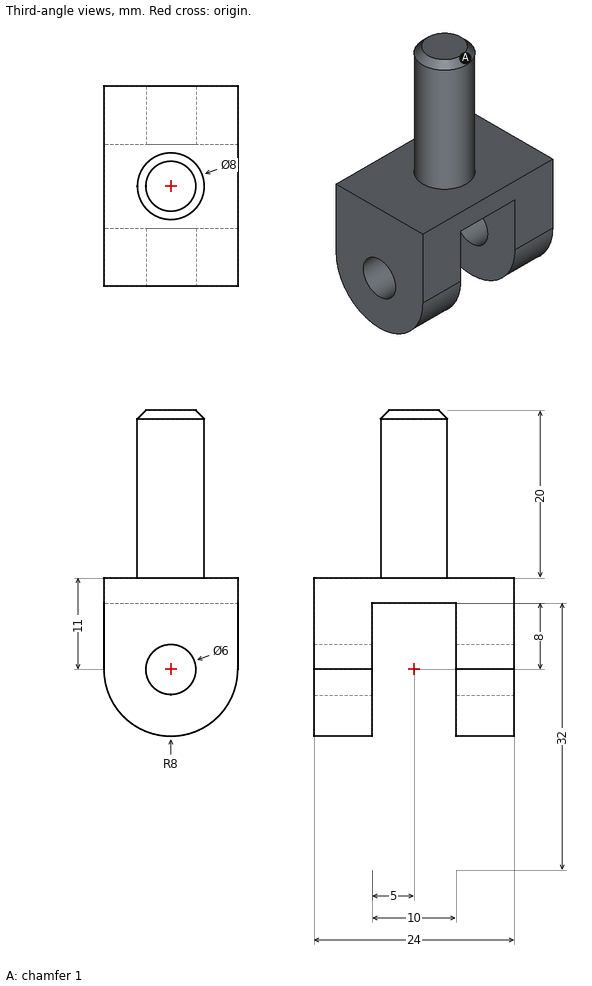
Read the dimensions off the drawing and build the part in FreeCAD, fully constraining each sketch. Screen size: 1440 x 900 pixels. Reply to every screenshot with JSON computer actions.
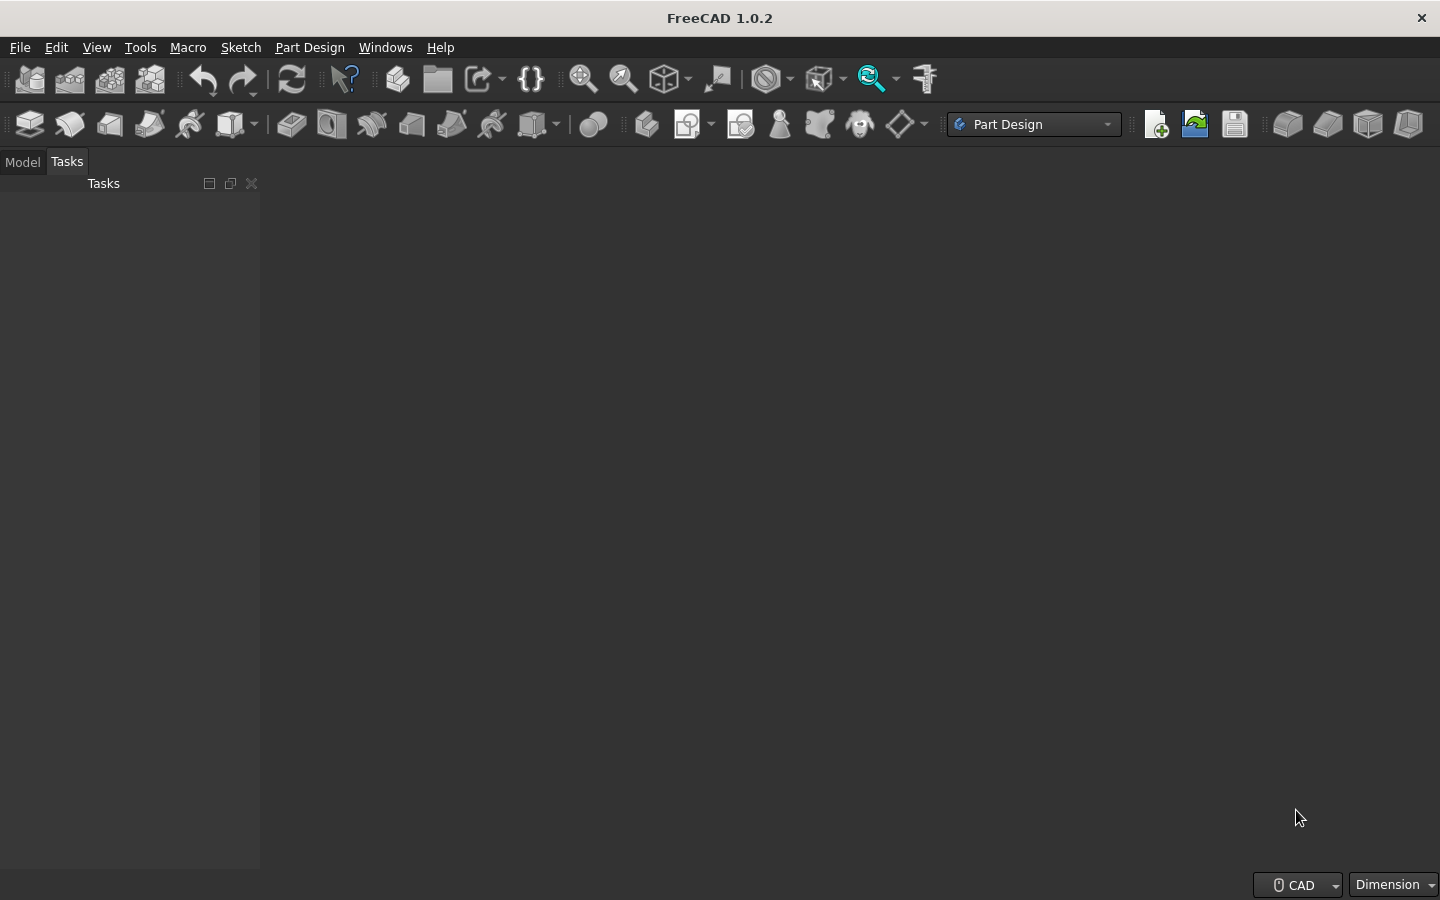
{"action": "left_click", "coordinate": [1156, 124]}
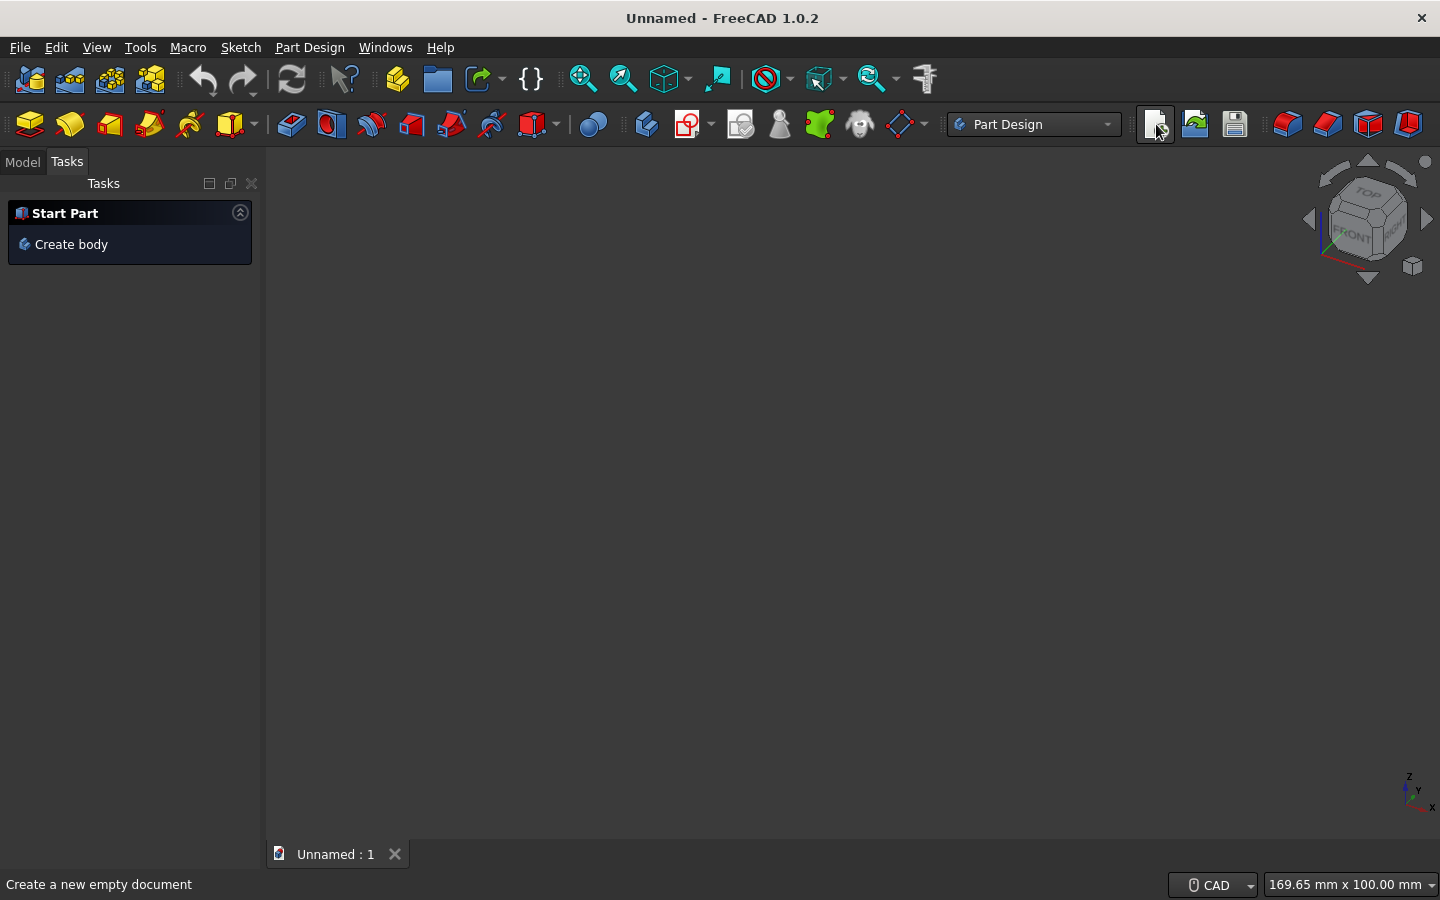
{"action": "left_click", "coordinate": [688, 124]}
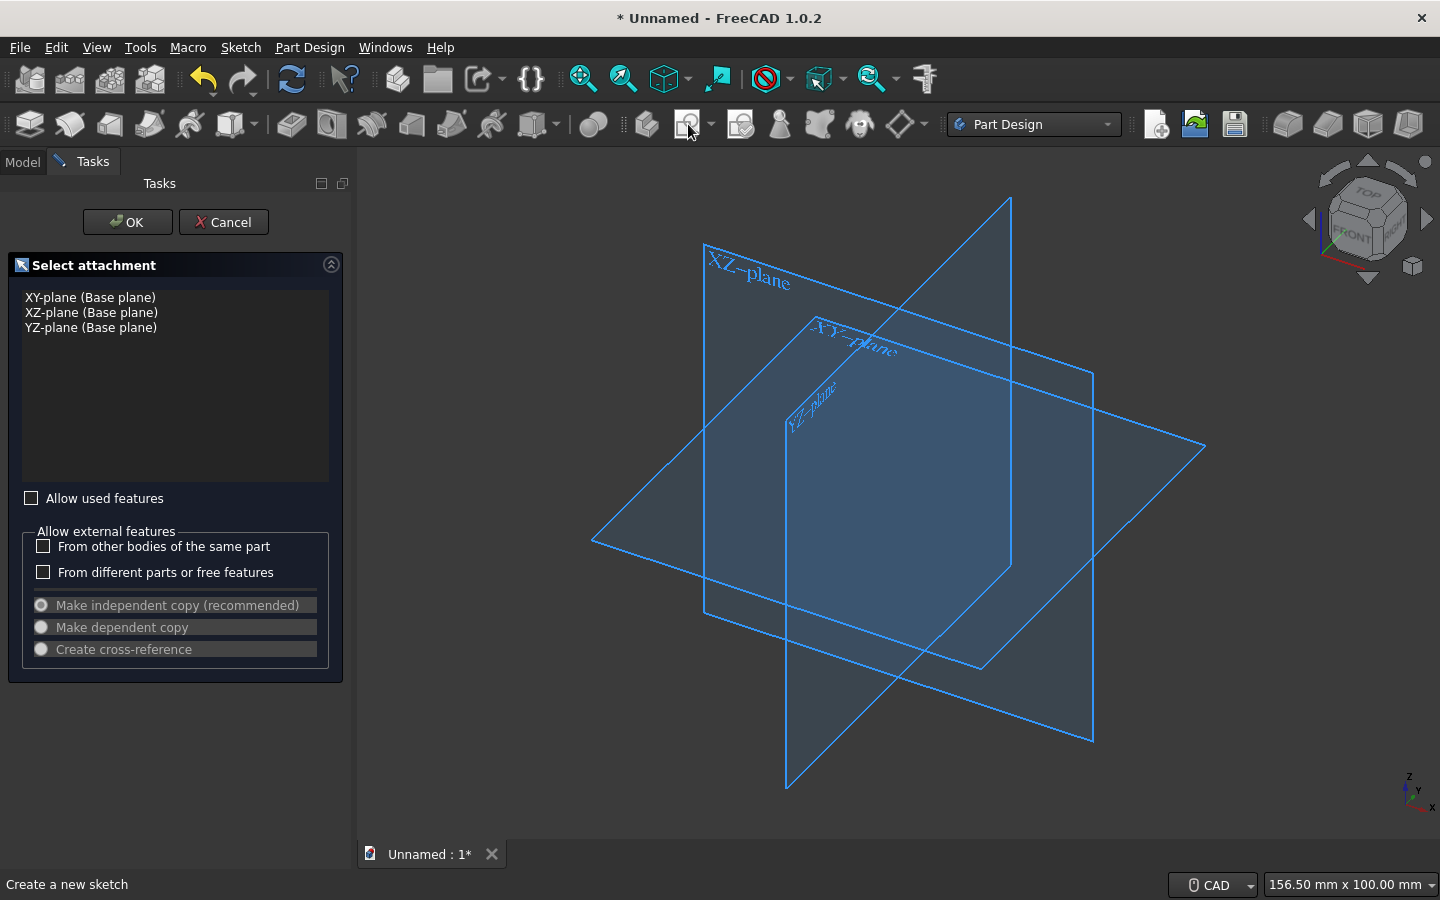
{"action": "left_click", "coordinate": [82, 312]}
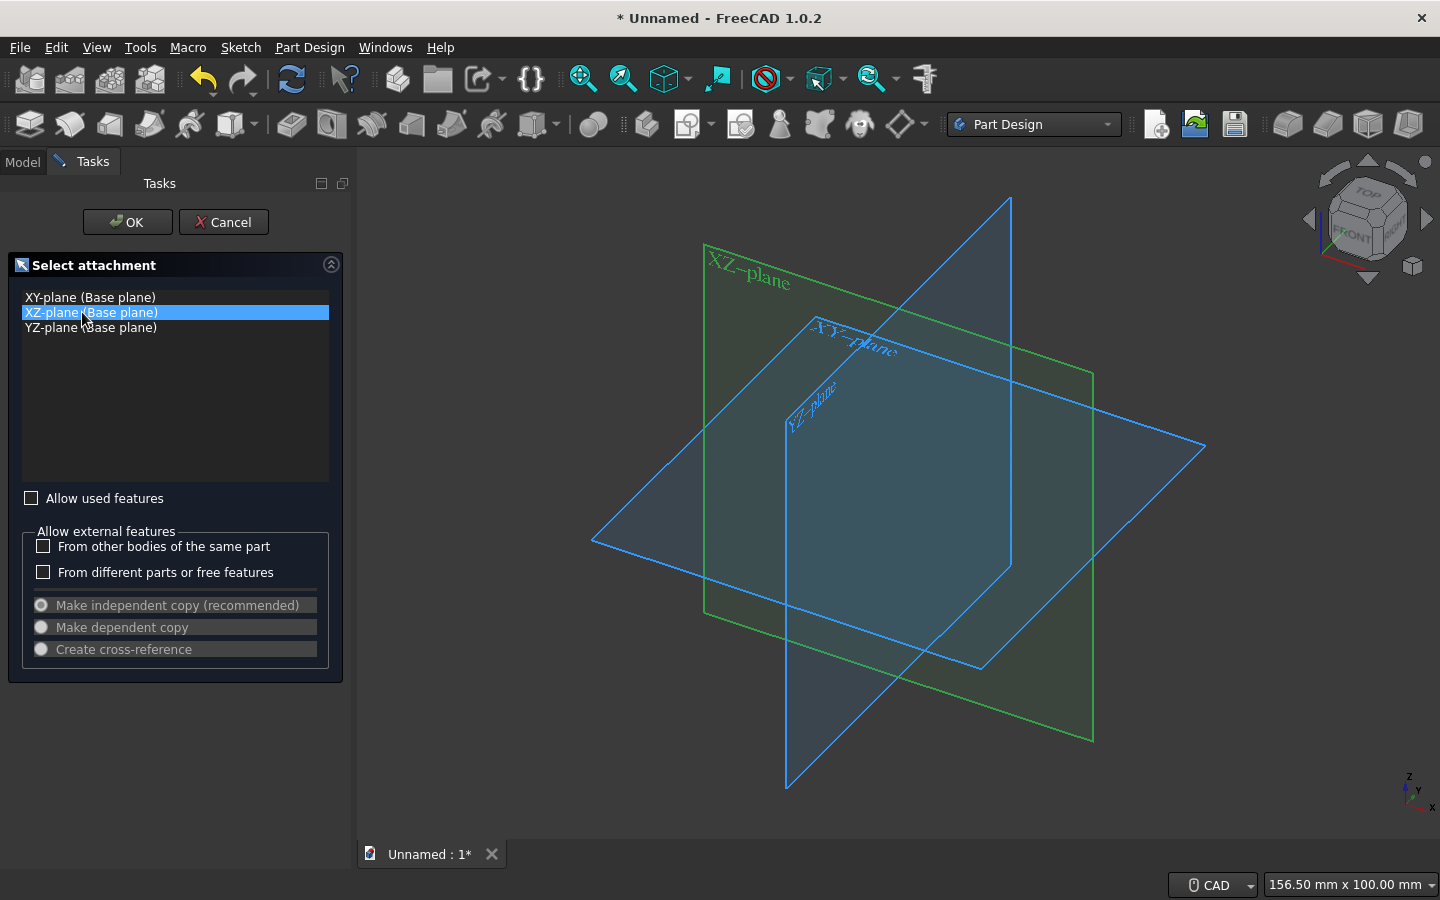
{"action": "left_click", "coordinate": [128, 222]}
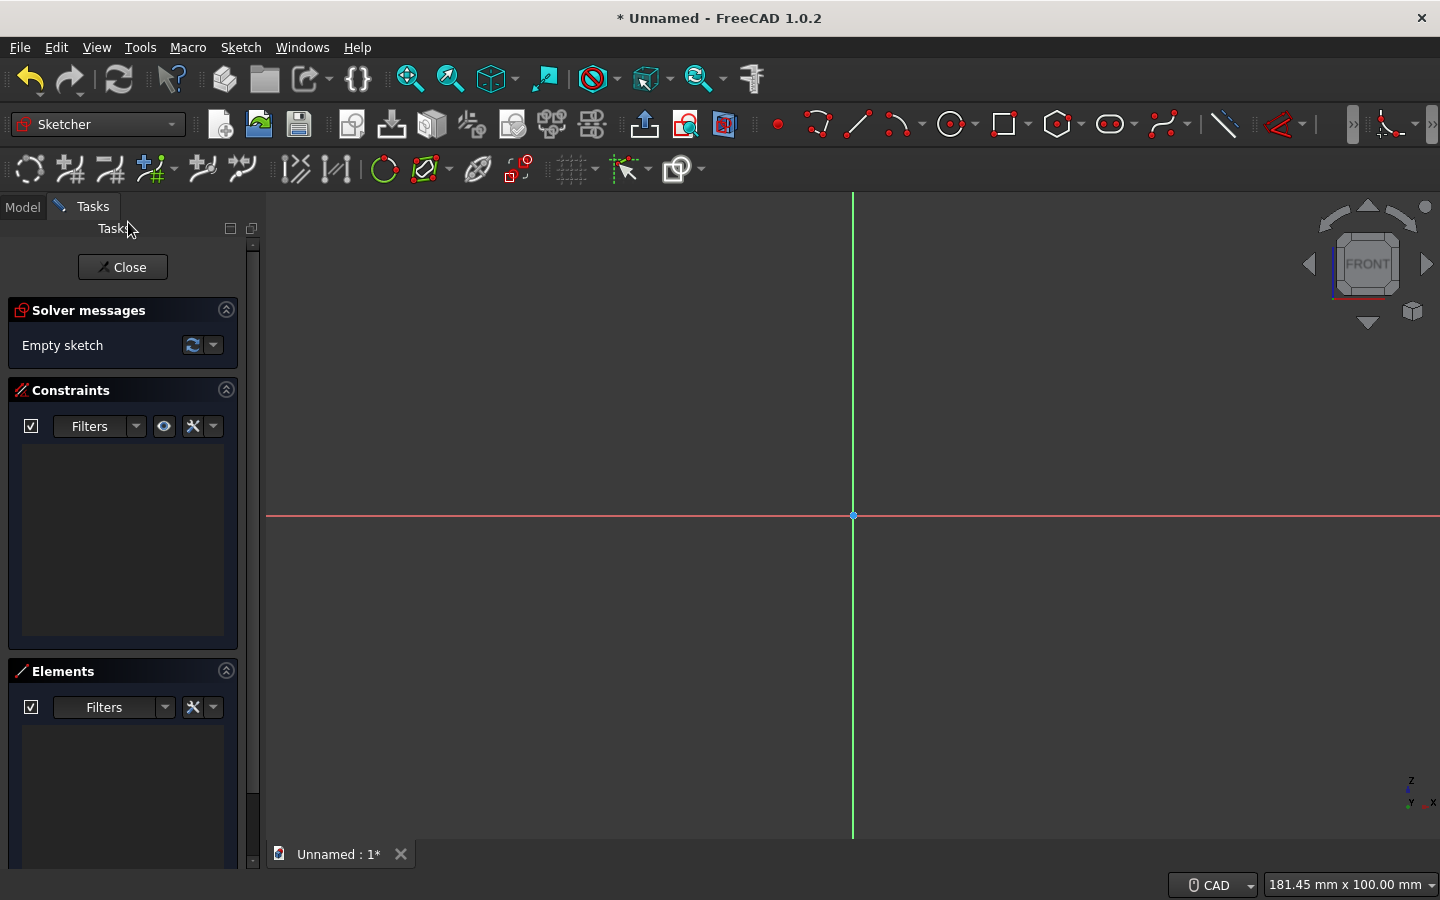
{"action": "scroll", "coordinate": [883, 502], "scroll_direction": "up", "scroll_amount": 6}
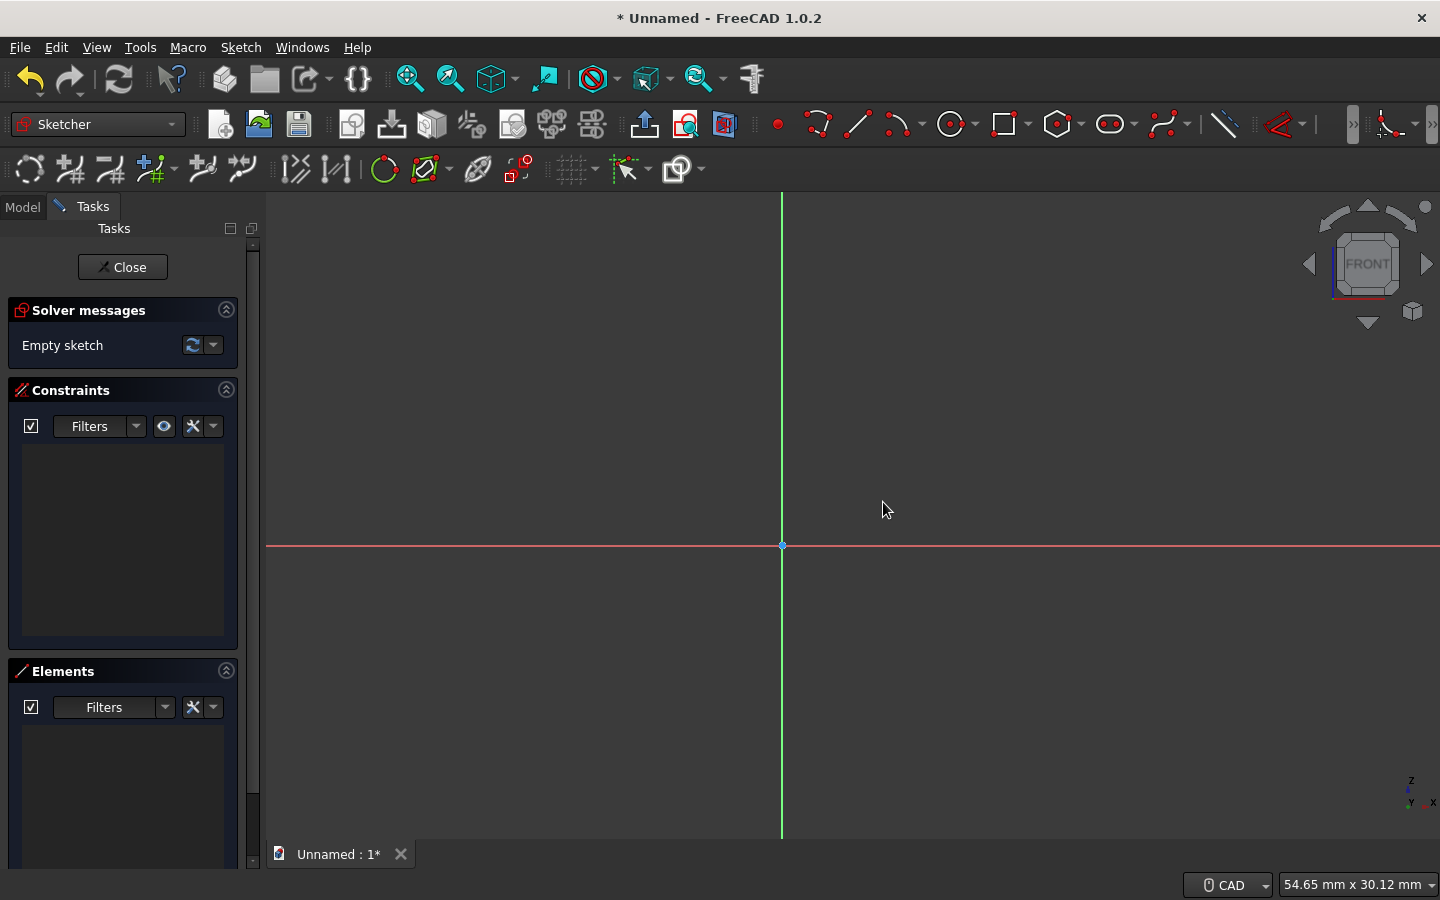
{"action": "left_click", "coordinate": [818, 124]}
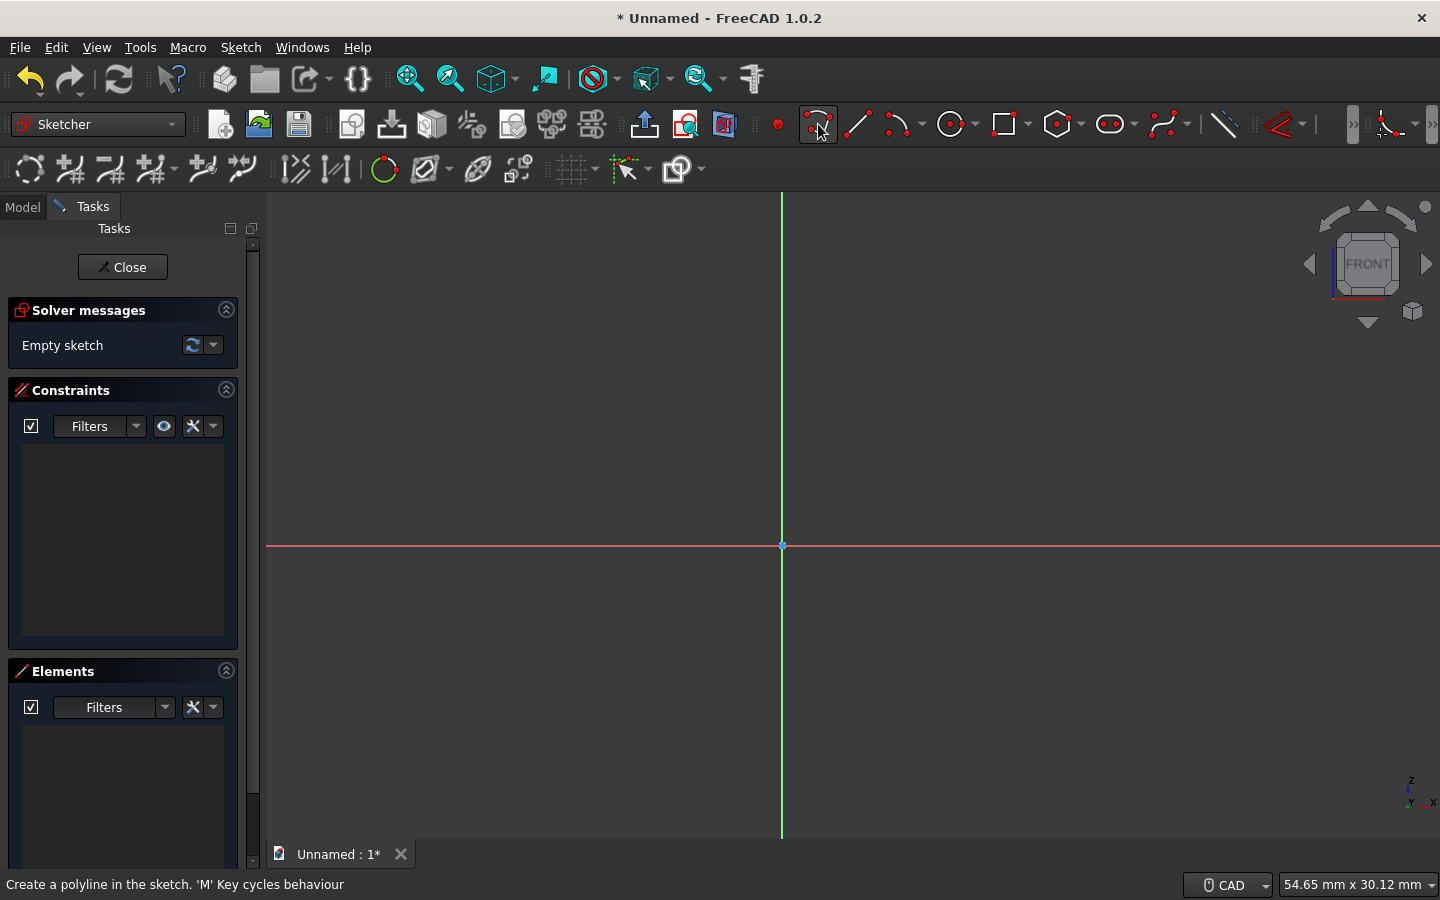
{"action": "left_click", "coordinate": [610, 546]}
{"action": "left_click", "coordinate": [610, 309]}
{"action": "left_click", "coordinate": [954, 309]}
{"action": "left_click", "coordinate": [954, 546]}
{"action": "right_click", "coordinate": [954, 546]}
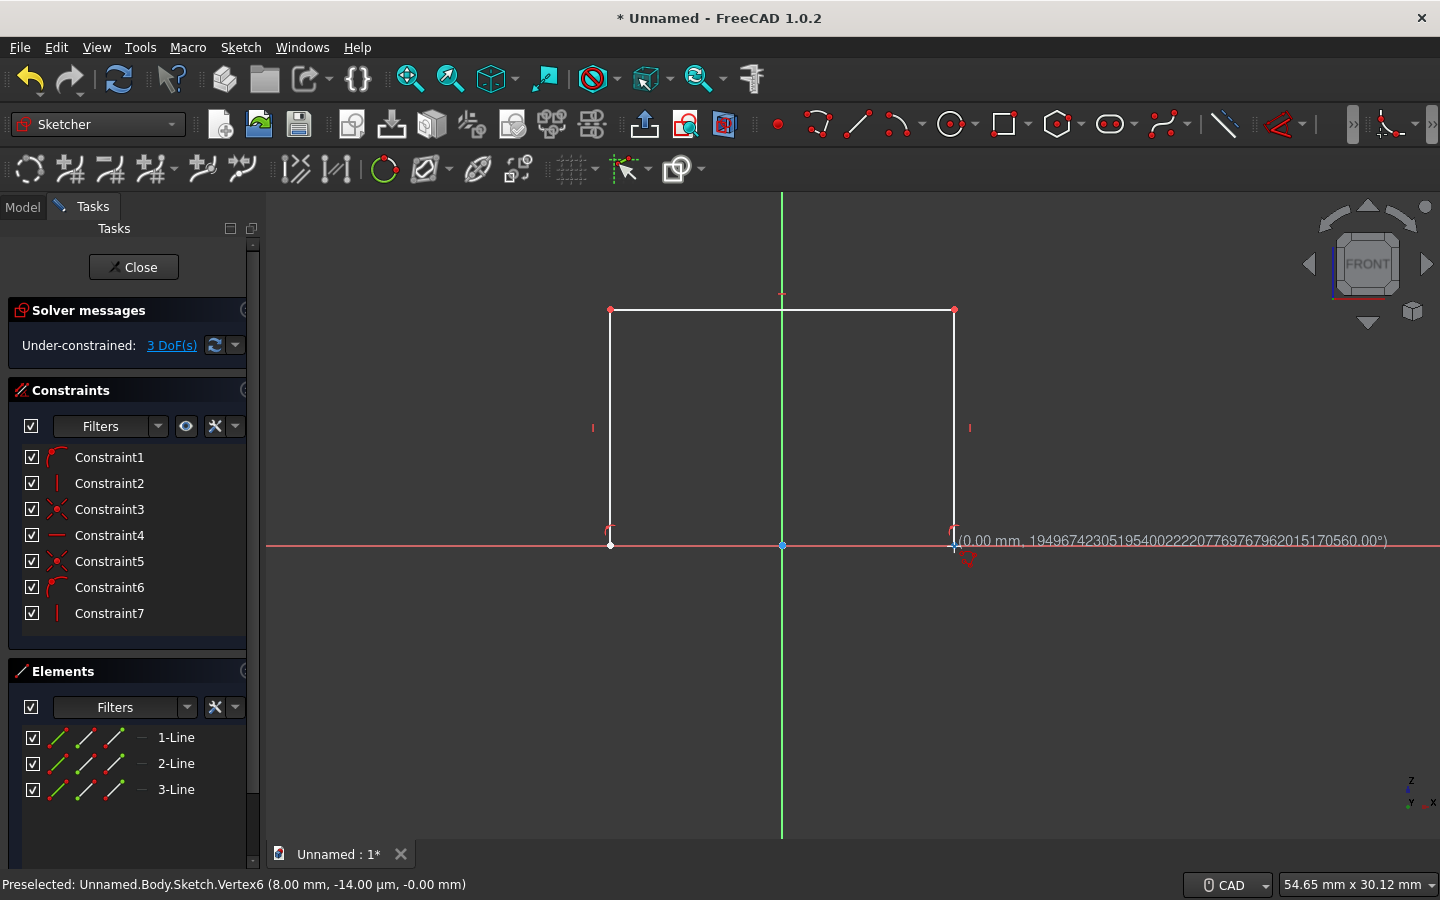
{"action": "key", "text": "g 3 a"}